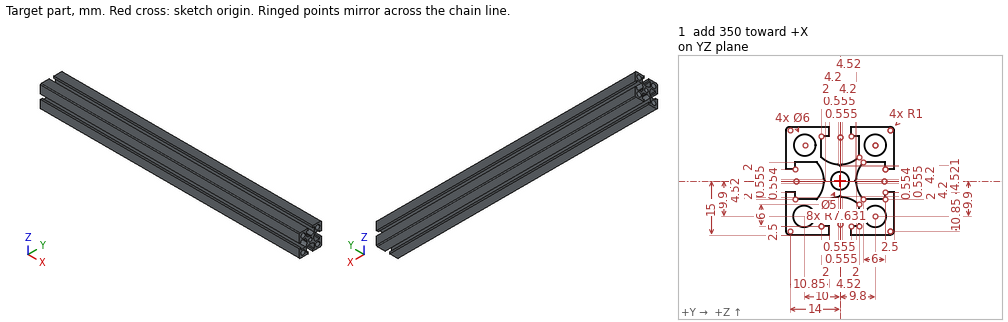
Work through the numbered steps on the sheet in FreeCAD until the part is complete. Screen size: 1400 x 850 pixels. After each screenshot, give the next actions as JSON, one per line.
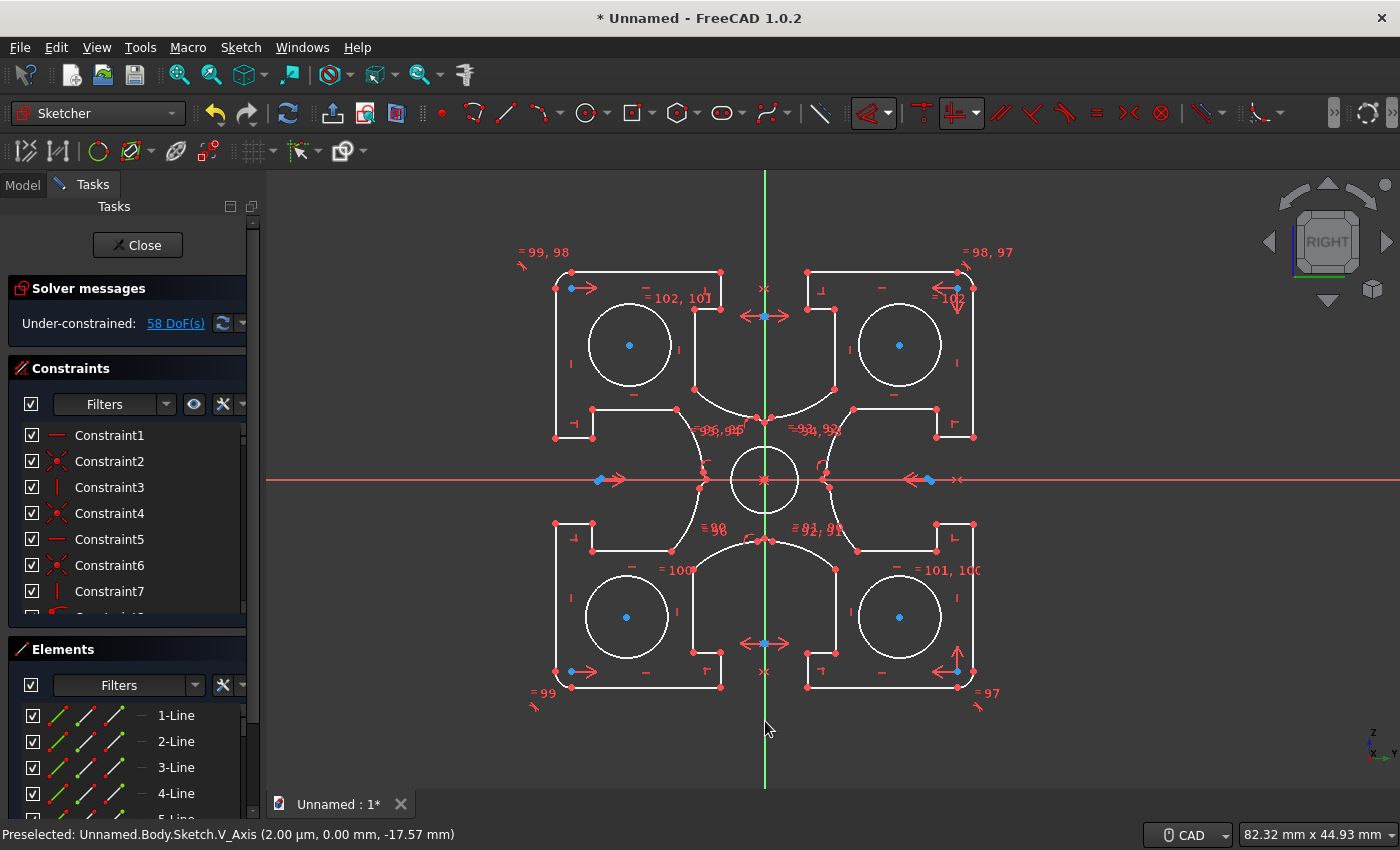
{"action": "left_click", "coordinate": [900, 617]}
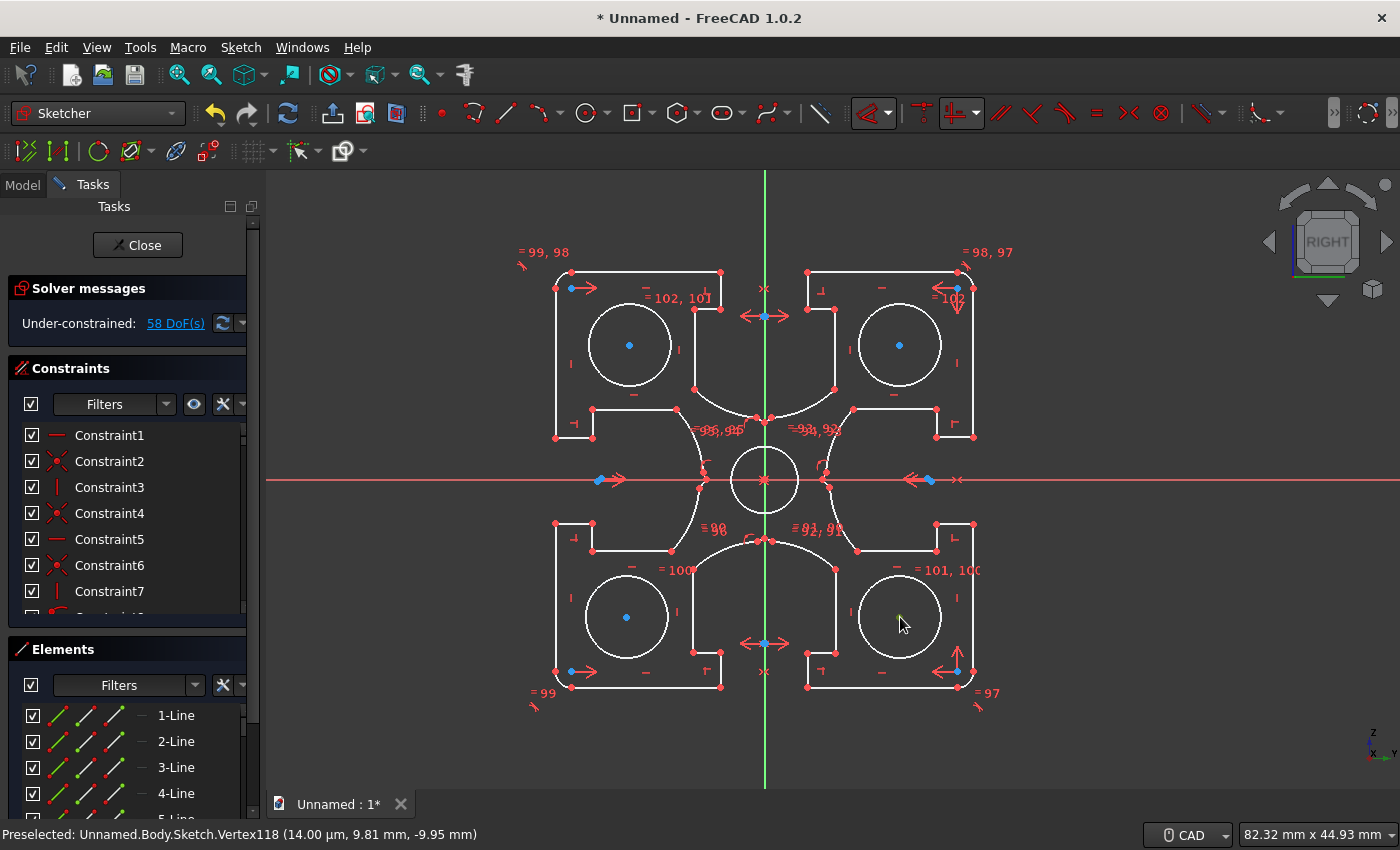
{"action": "left_click", "coordinate": [900, 345]}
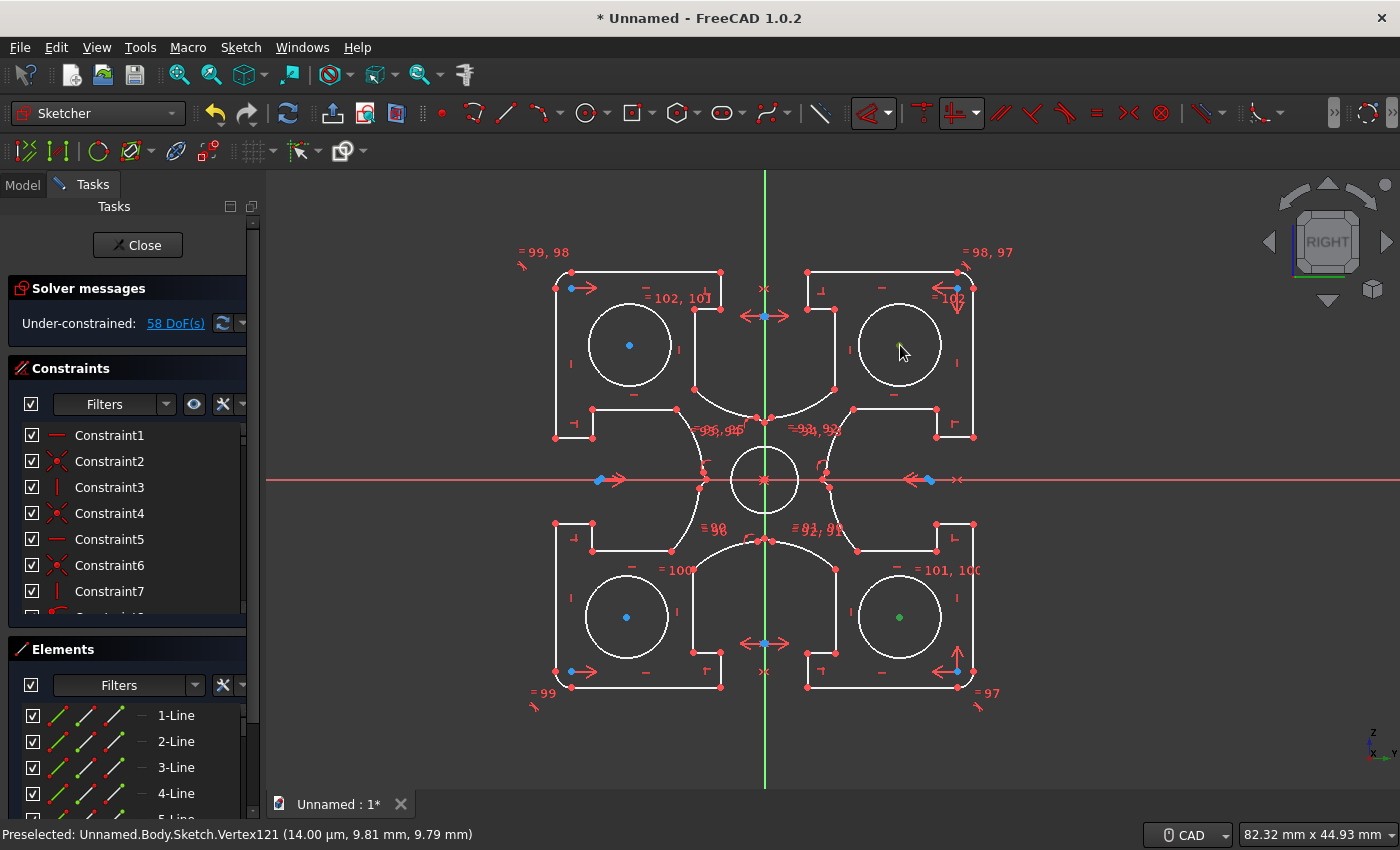
{"action": "left_click", "coordinate": [361, 480]}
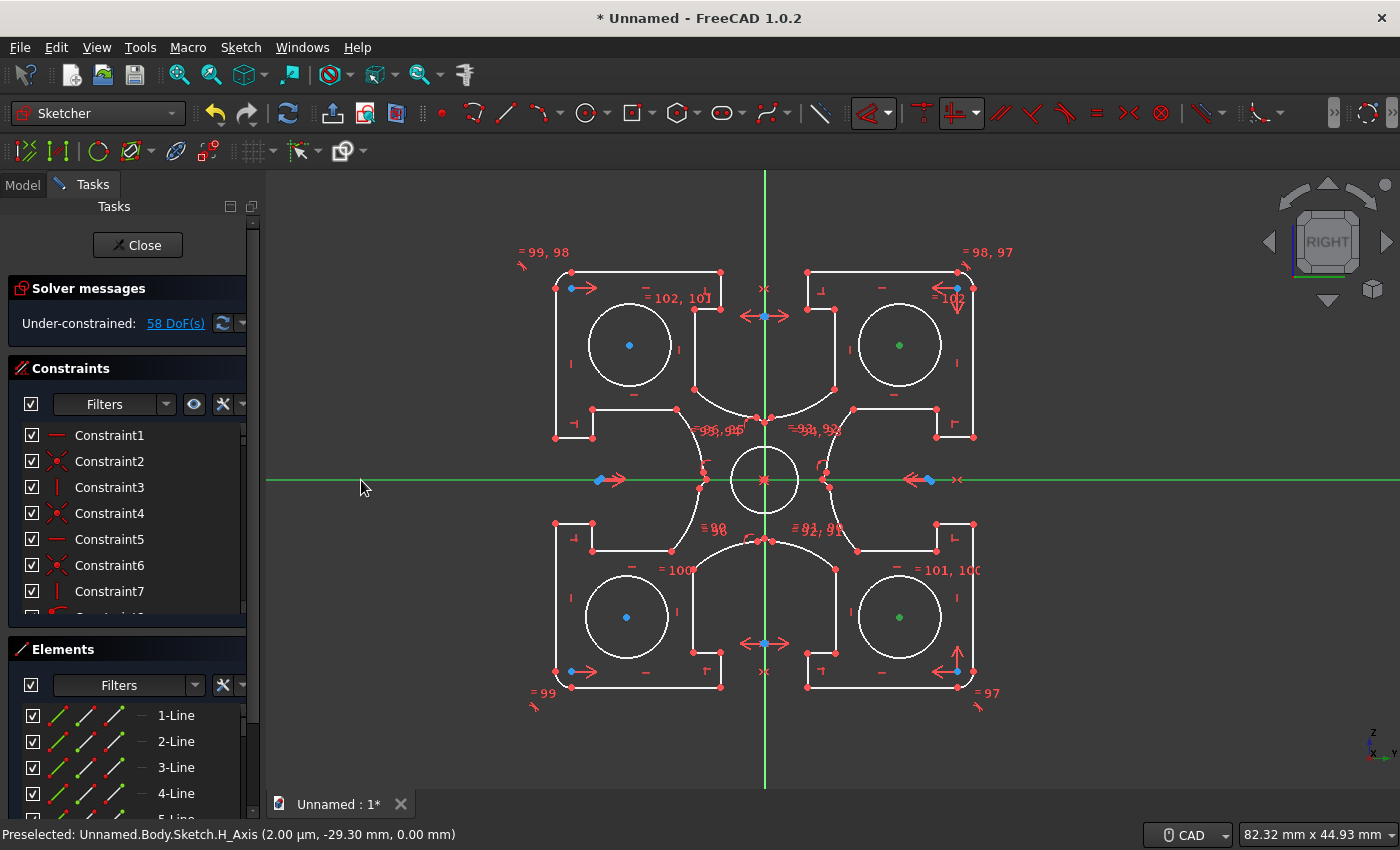
{"action": "left_click", "coordinate": [1130, 114]}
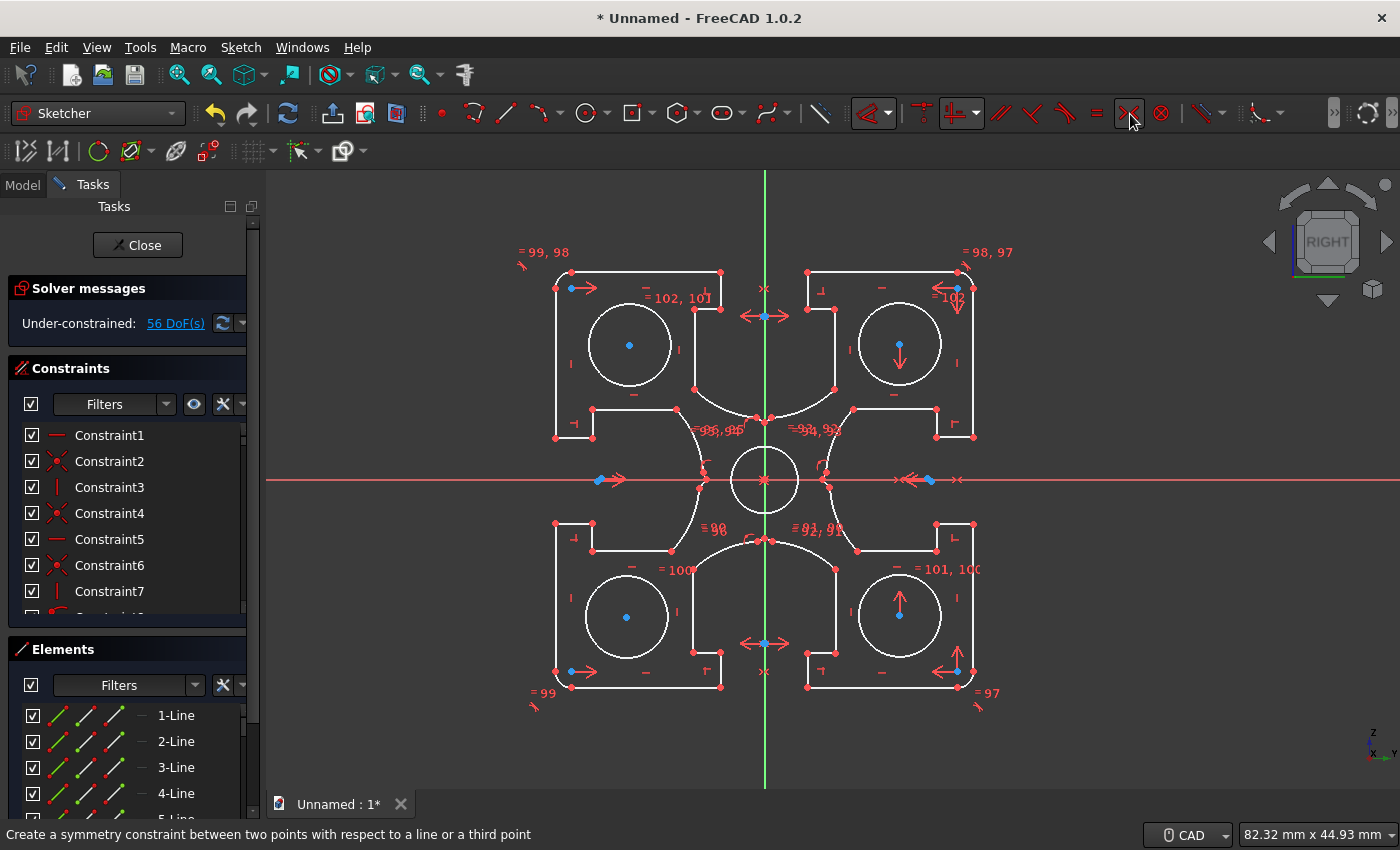
{"action": "left_click", "coordinate": [630, 345]}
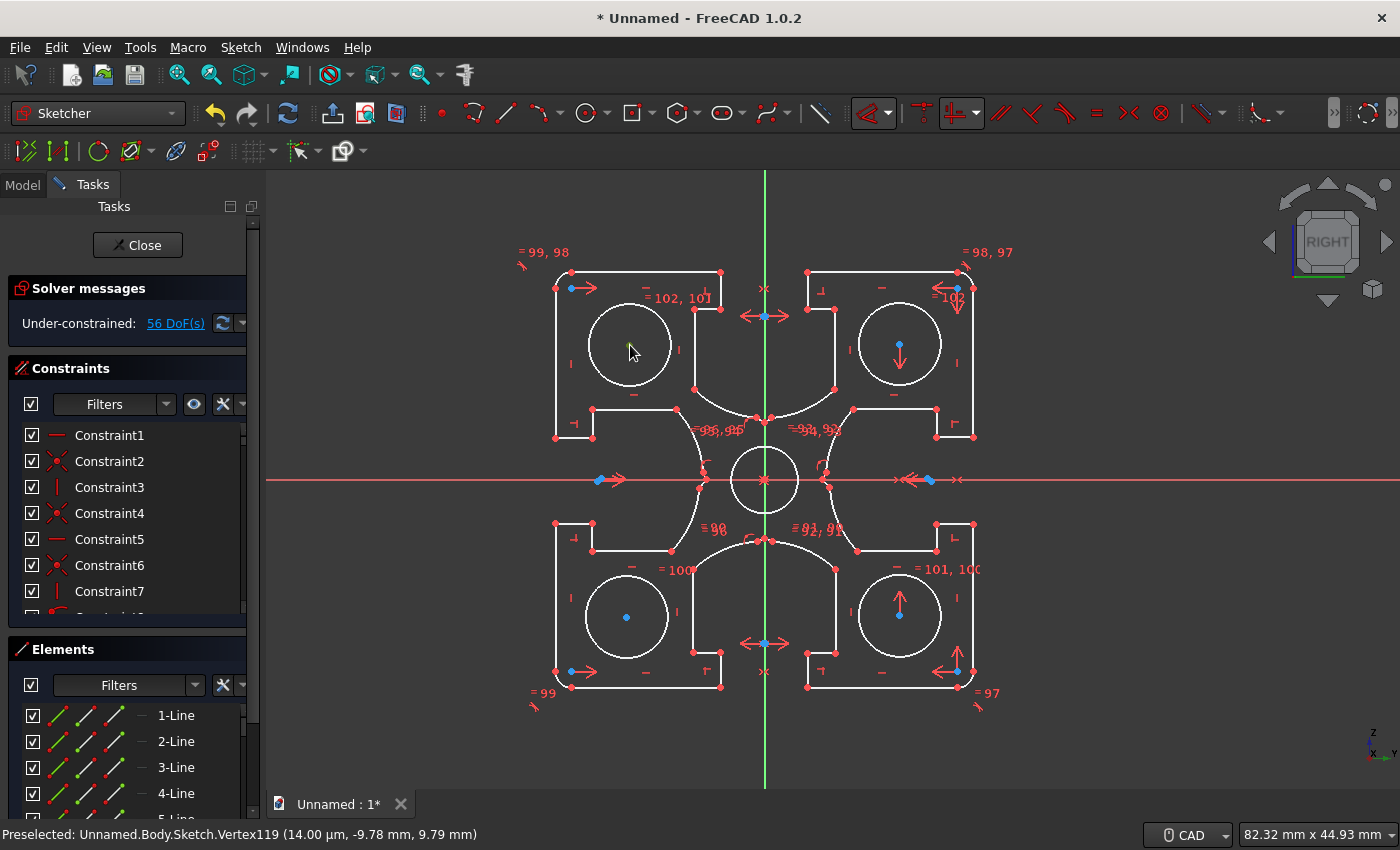
{"action": "left_click", "coordinate": [900, 344]}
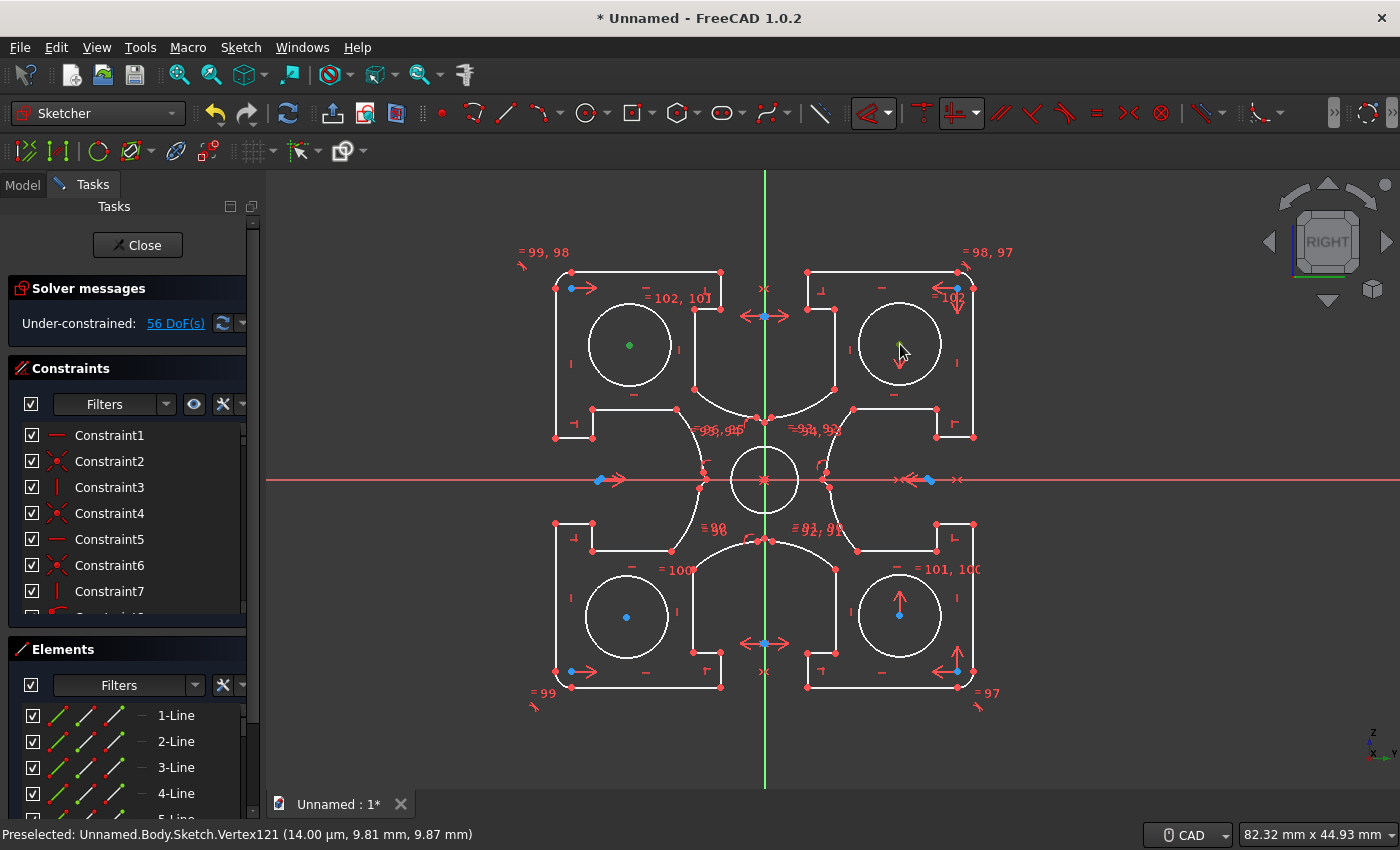
{"action": "left_click", "coordinate": [765, 721]}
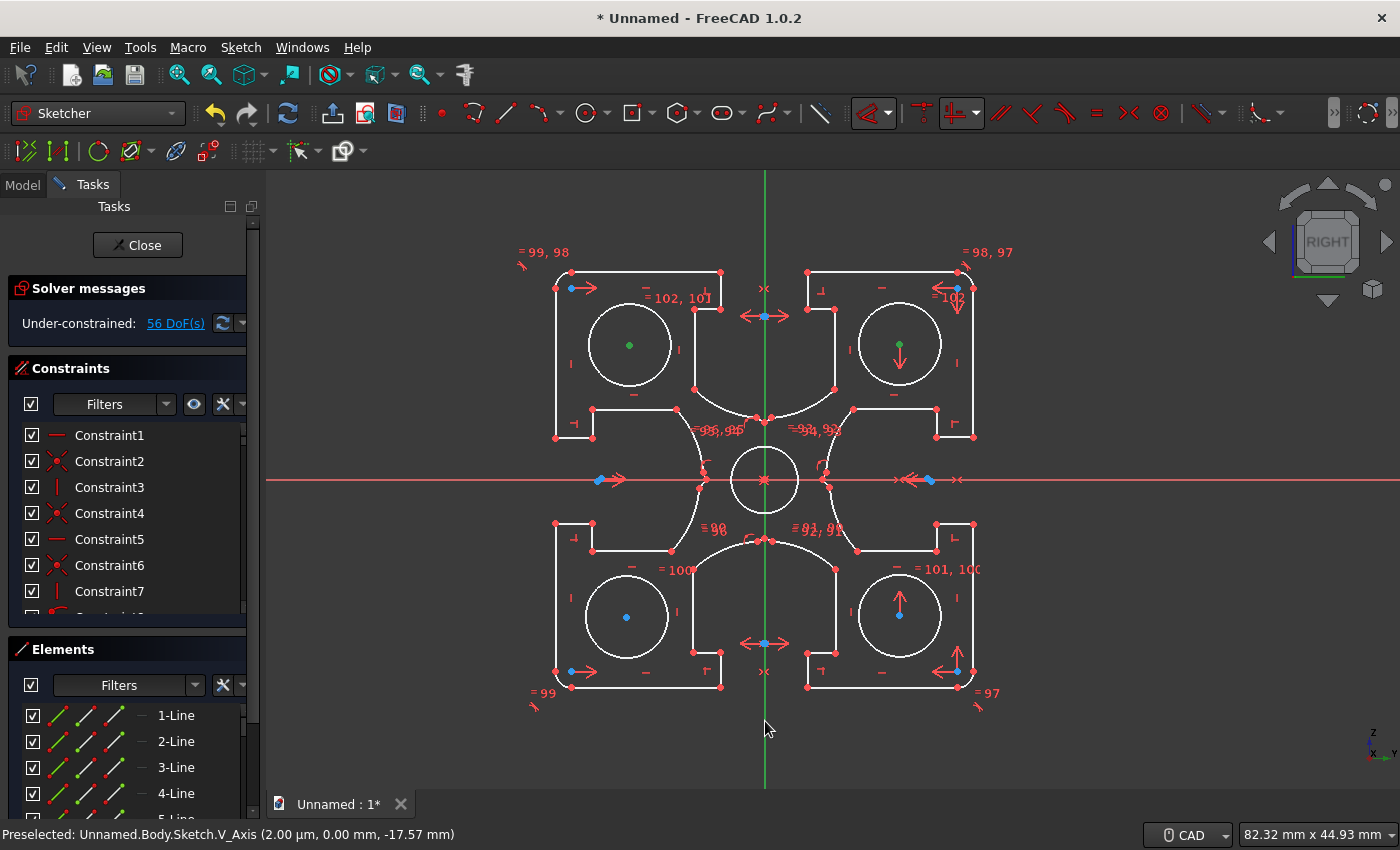
{"action": "key", "text": "s"}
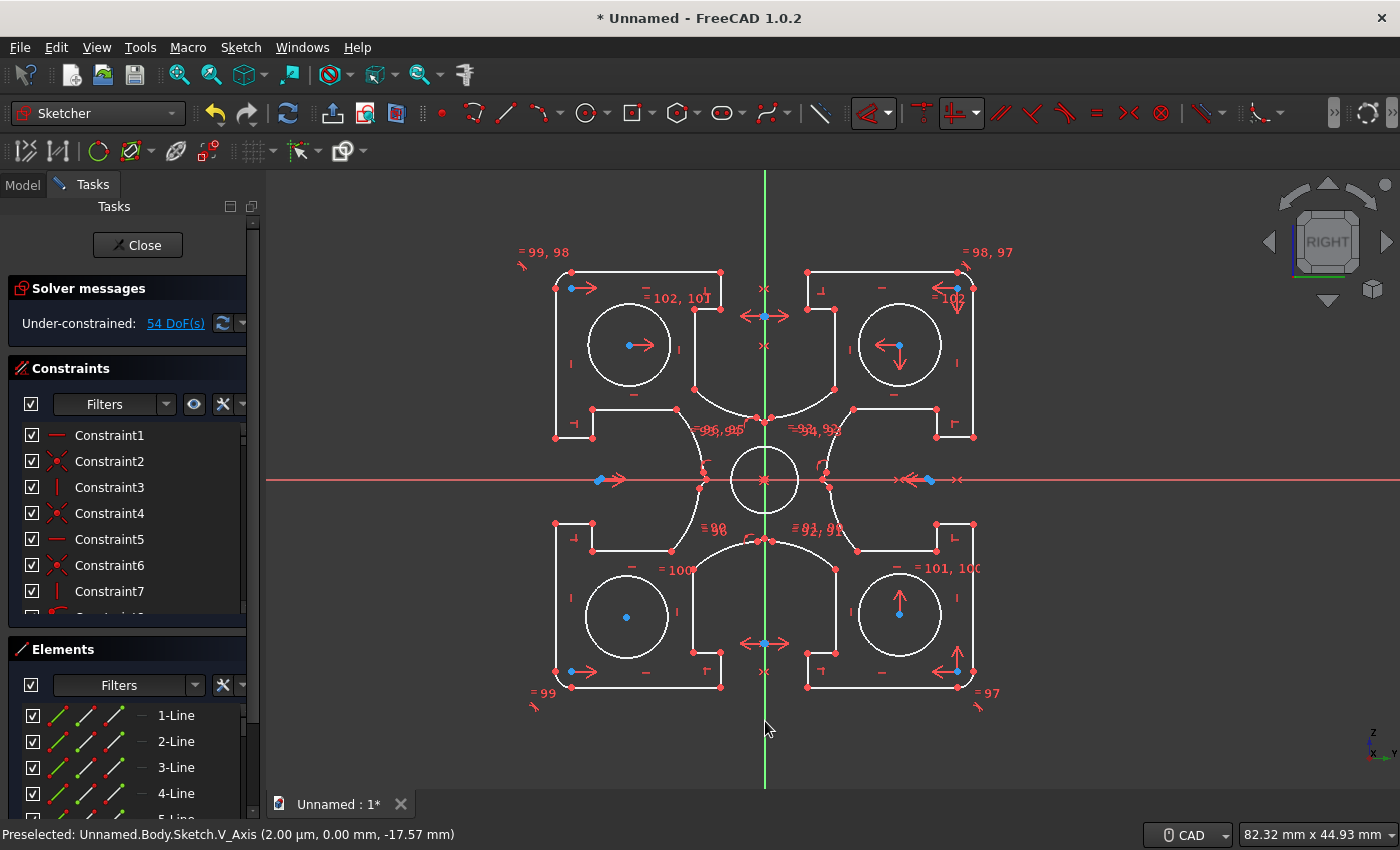
{"action": "left_click", "coordinate": [693, 653]}